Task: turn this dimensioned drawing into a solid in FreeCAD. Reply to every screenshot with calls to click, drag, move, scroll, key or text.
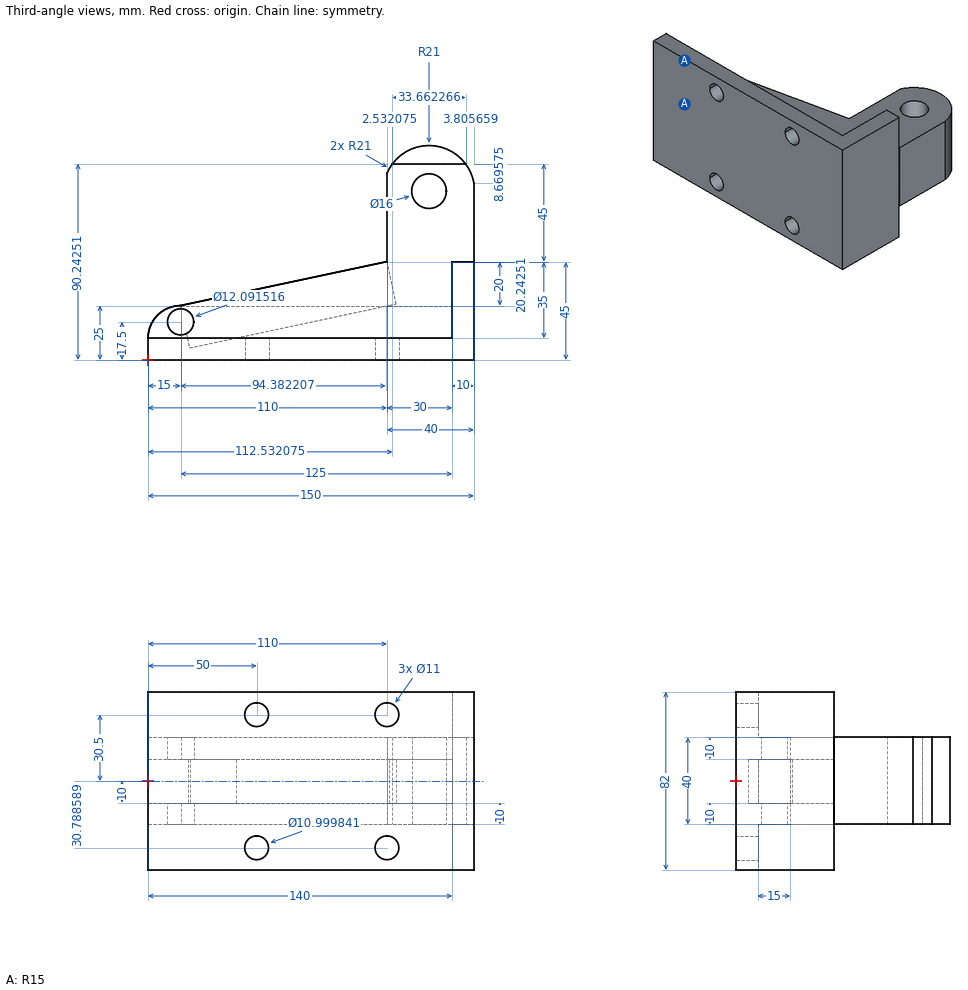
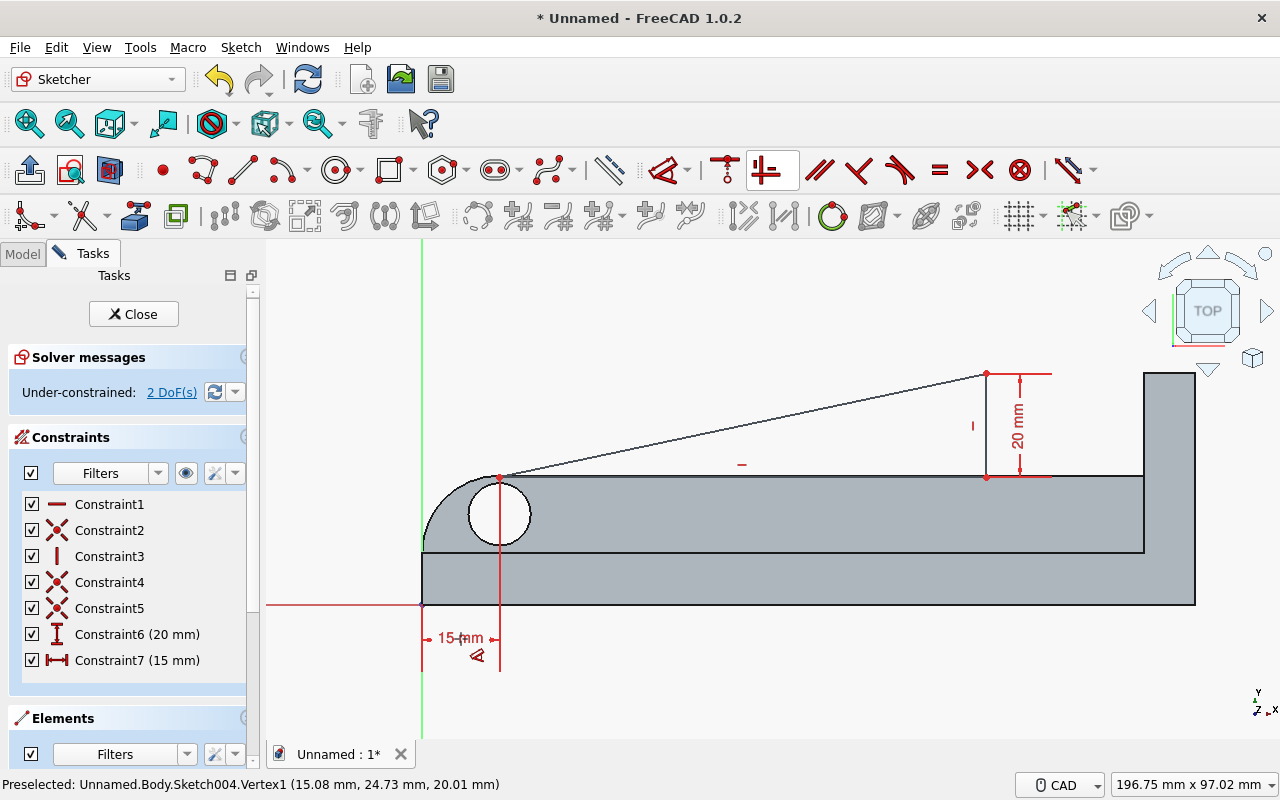
click(500, 477)
click(388, 541)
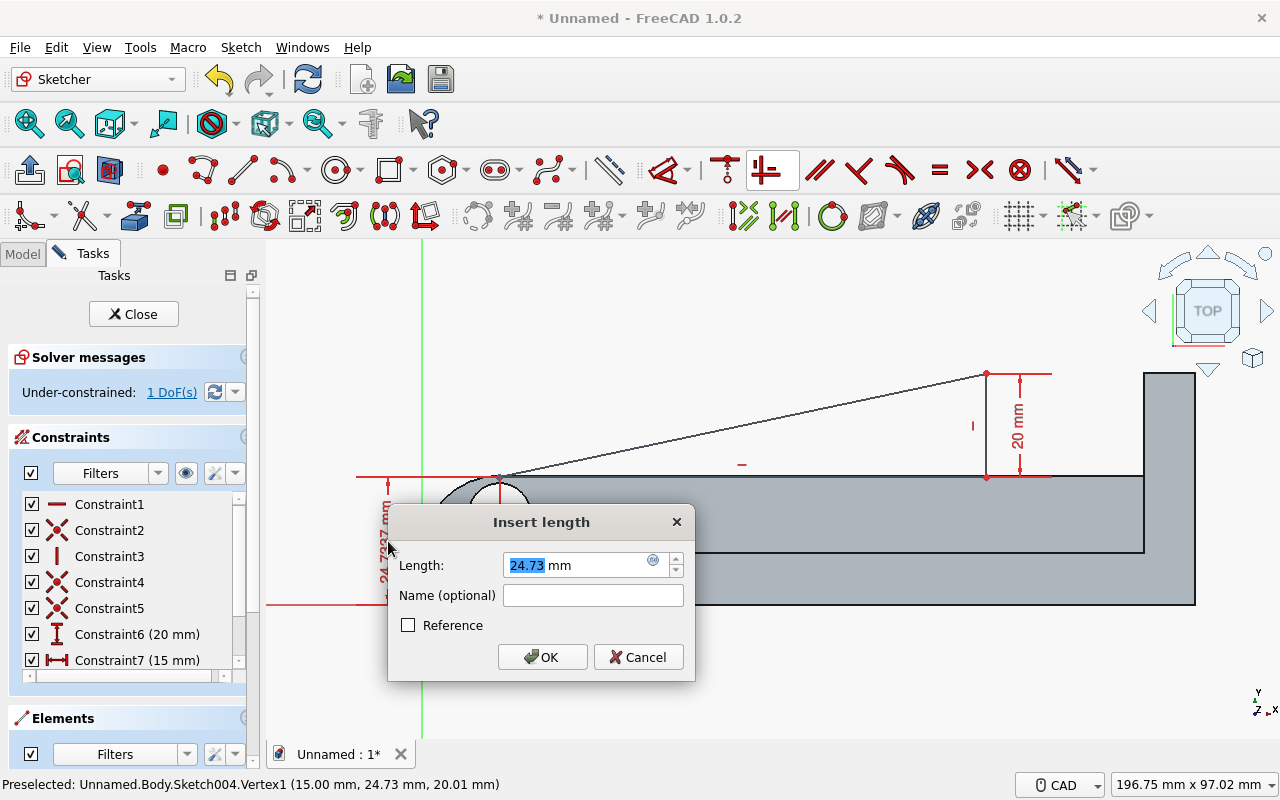
text(25)
key(Return)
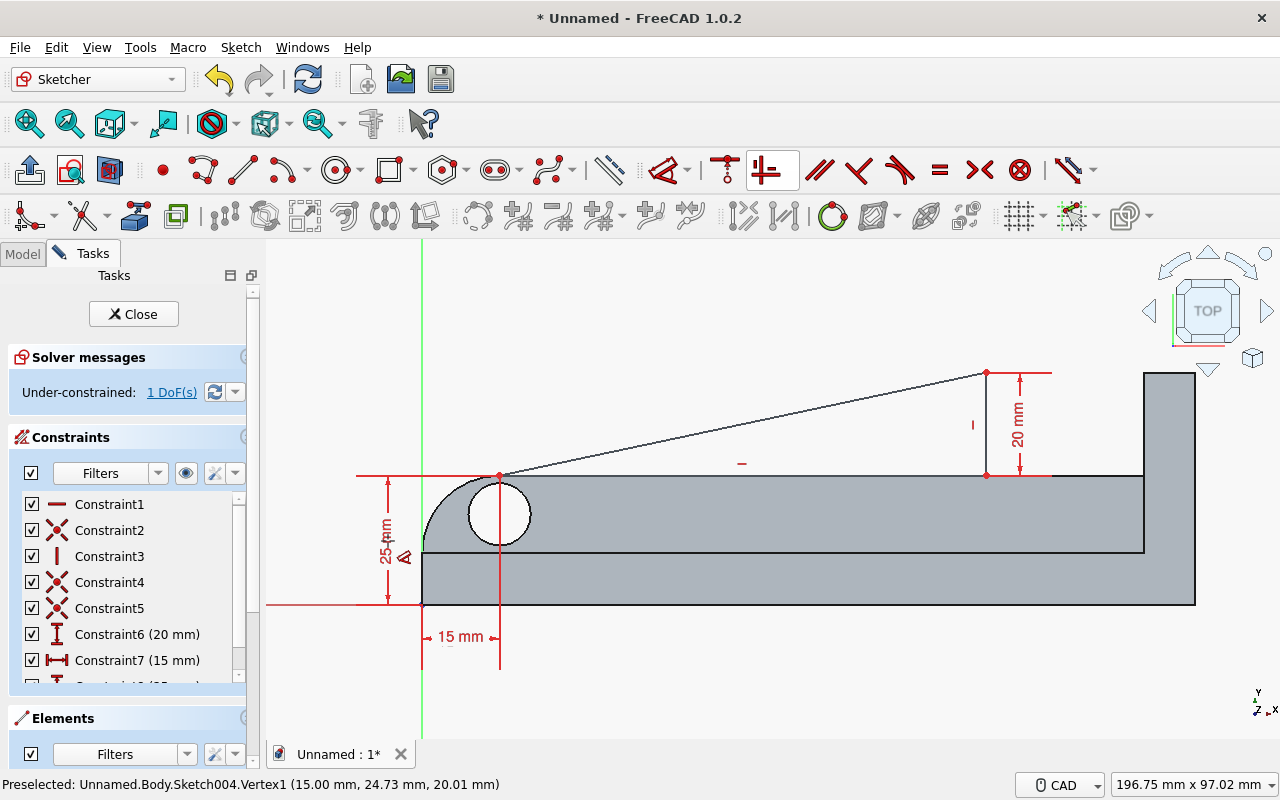
click(645, 476)
click(743, 442)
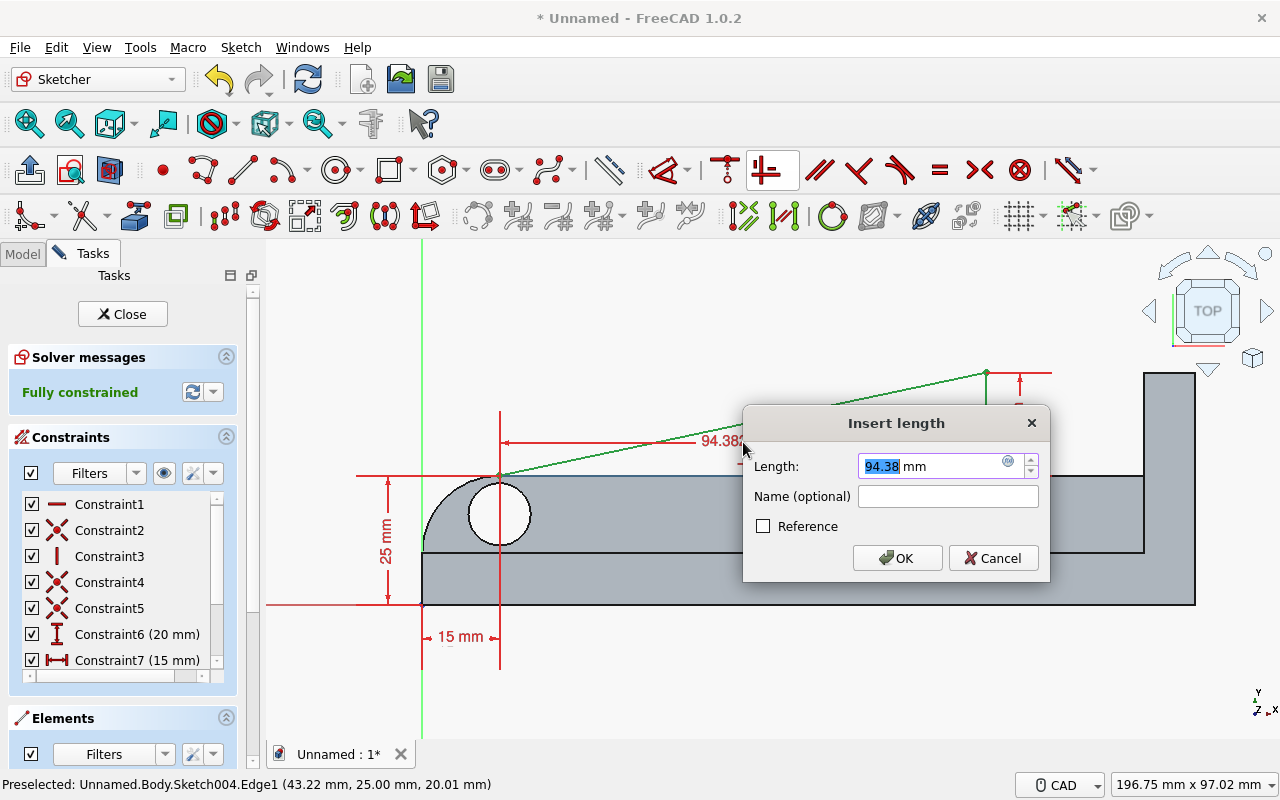
text(94.382207)
key(Return)
key(Escape)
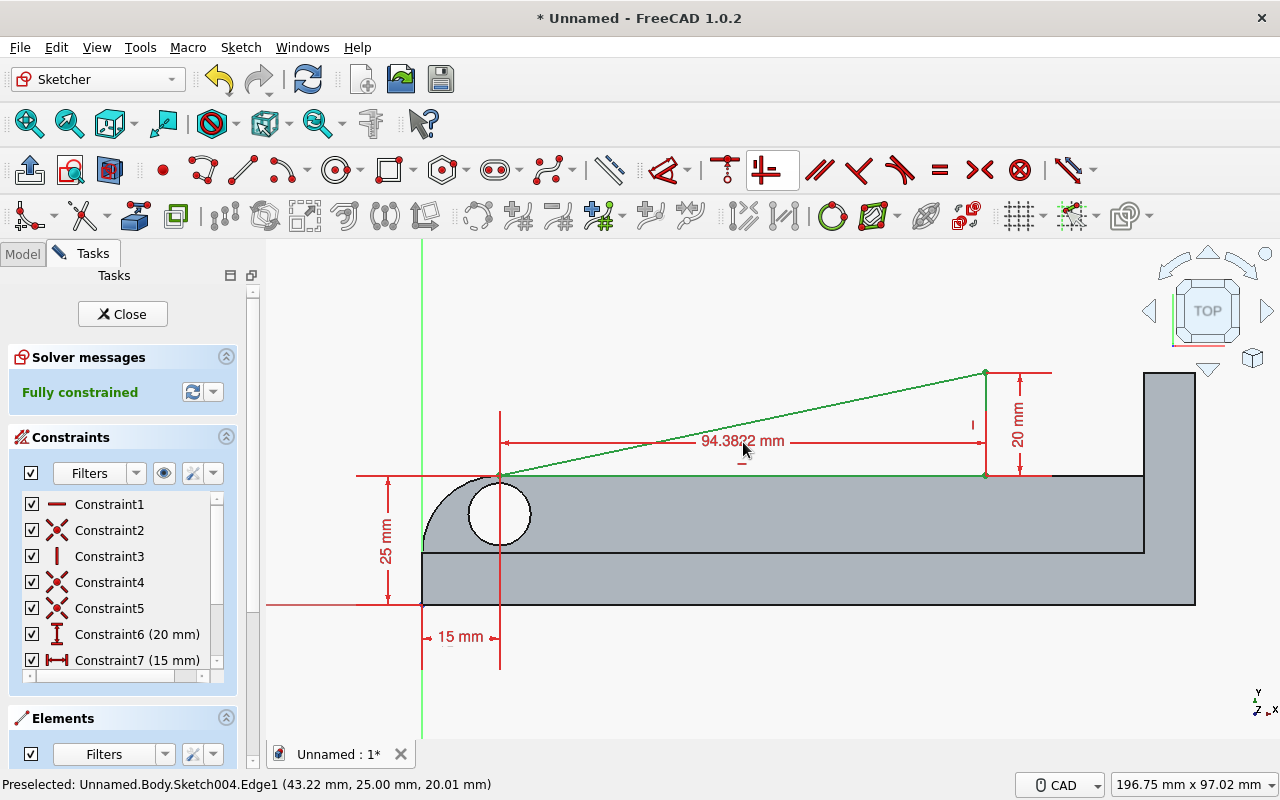
click(123, 314)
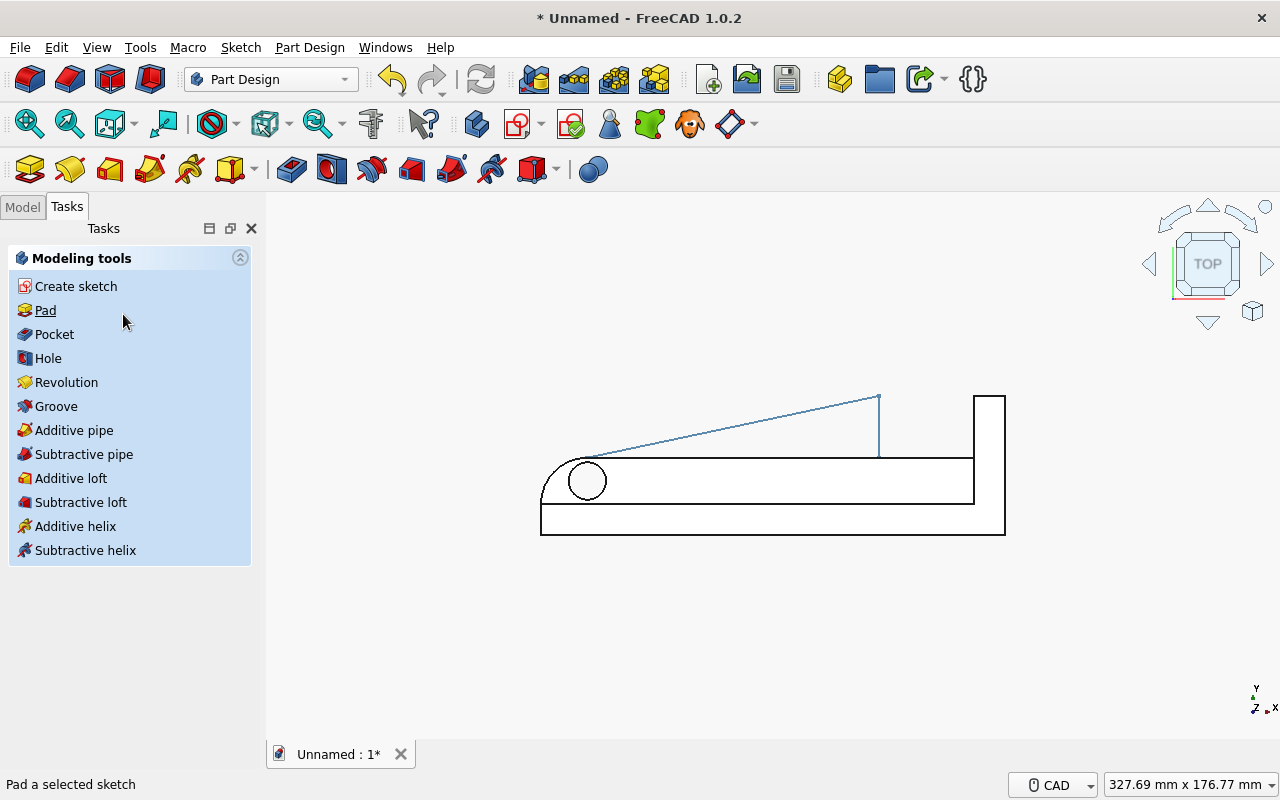
click(30, 170)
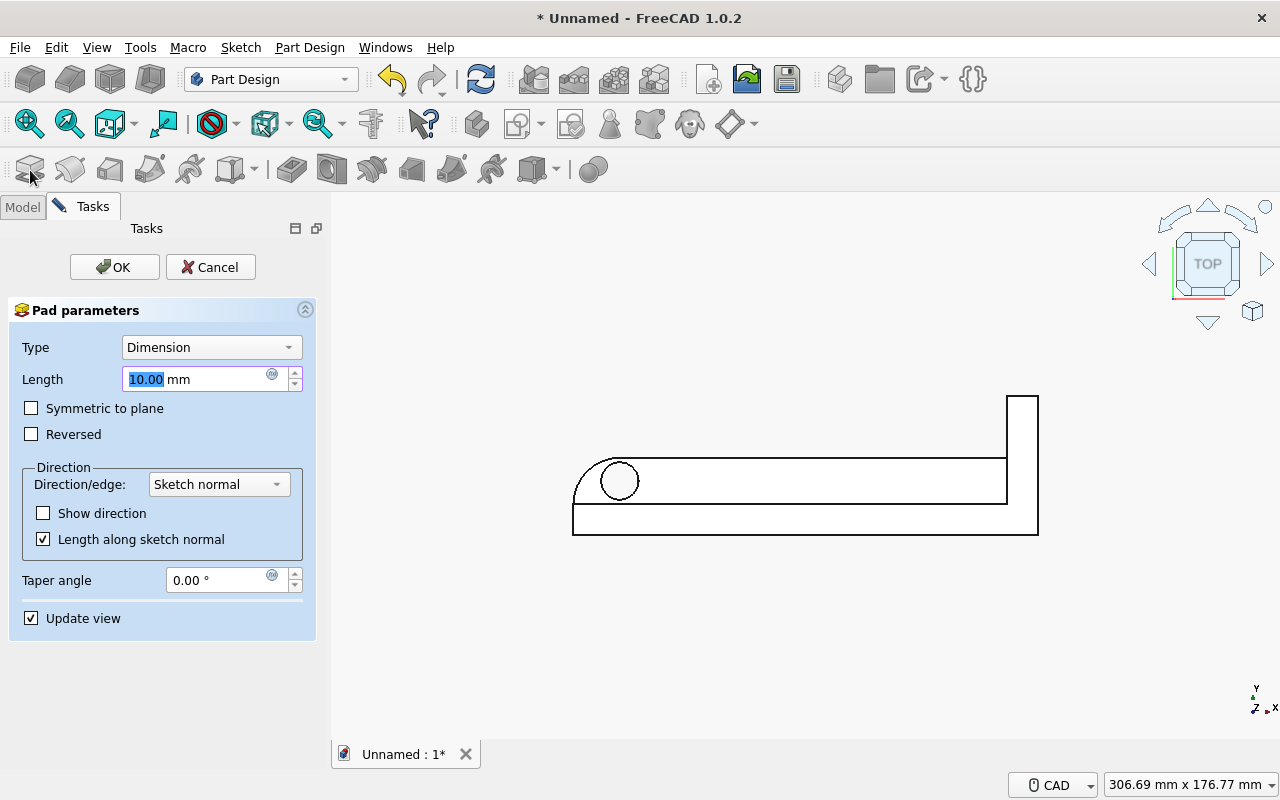
text(10)
key(Tab)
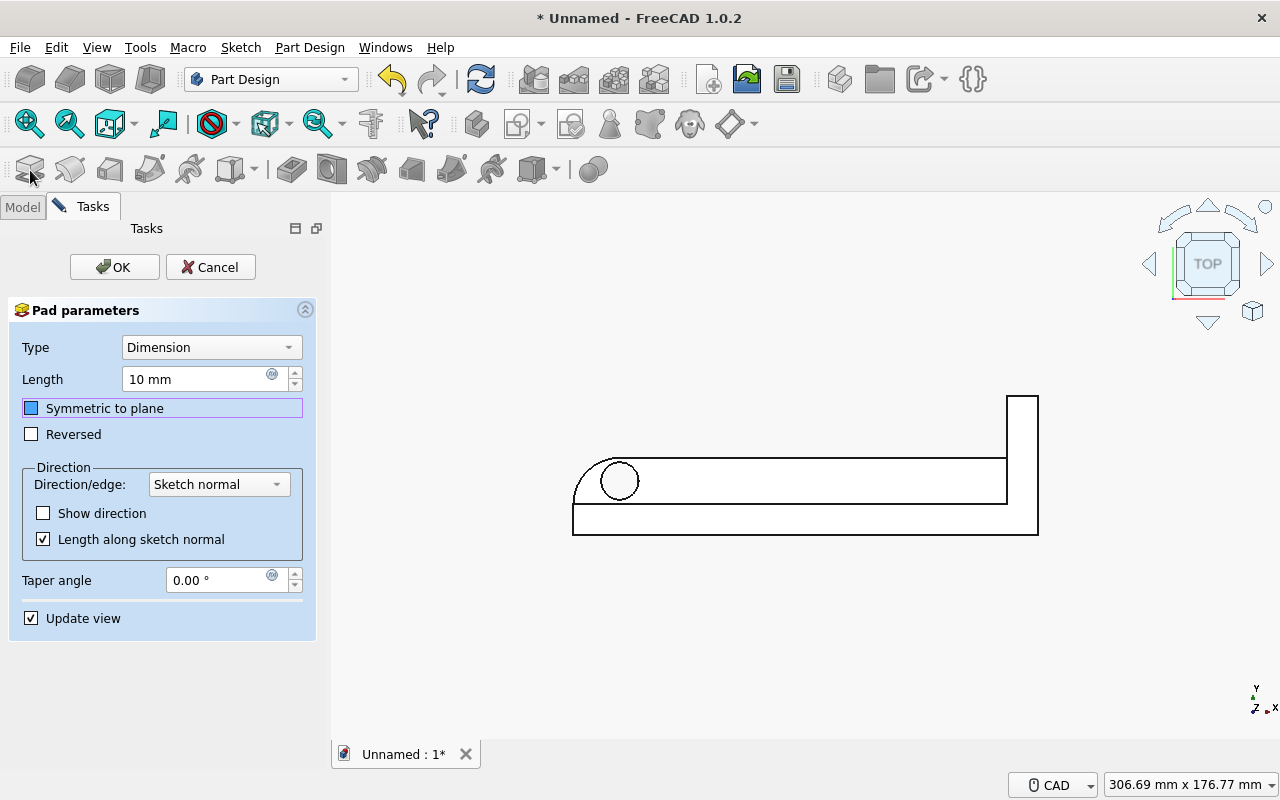
click(30, 434)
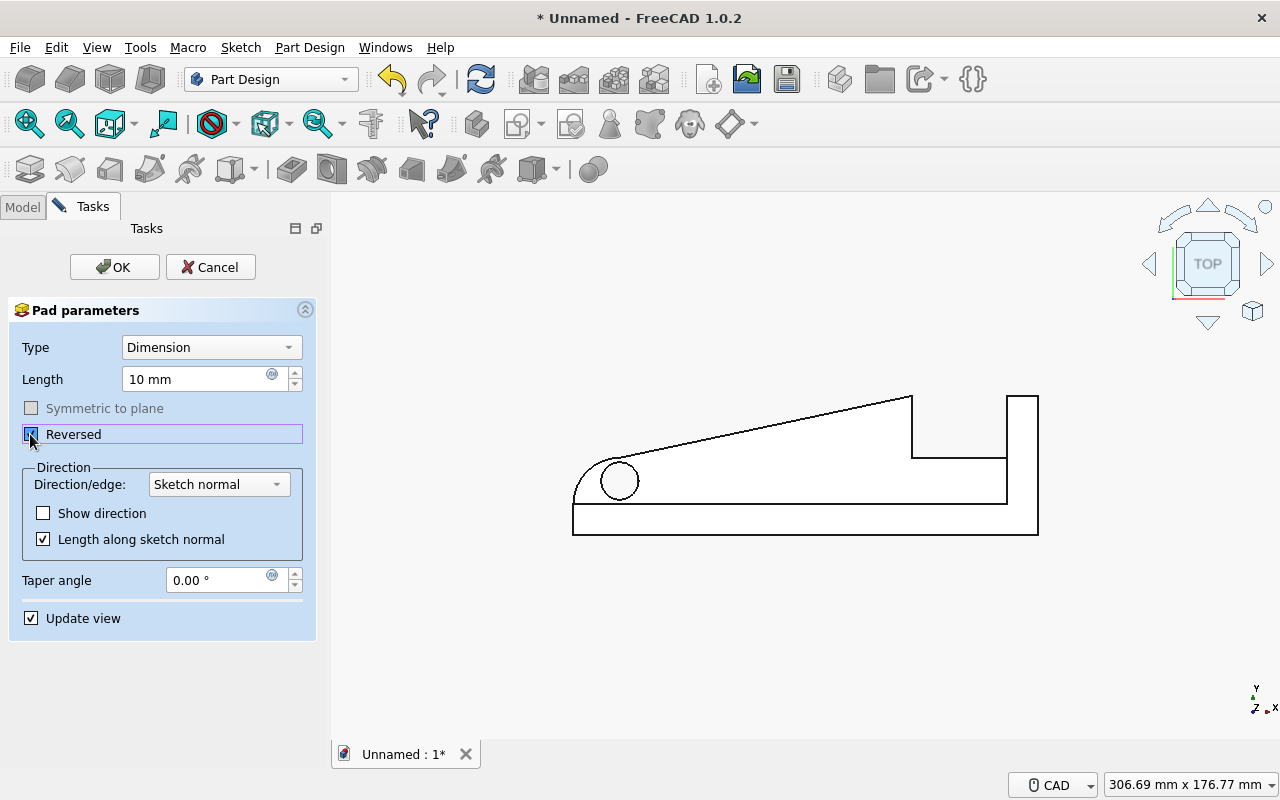
click(115, 267)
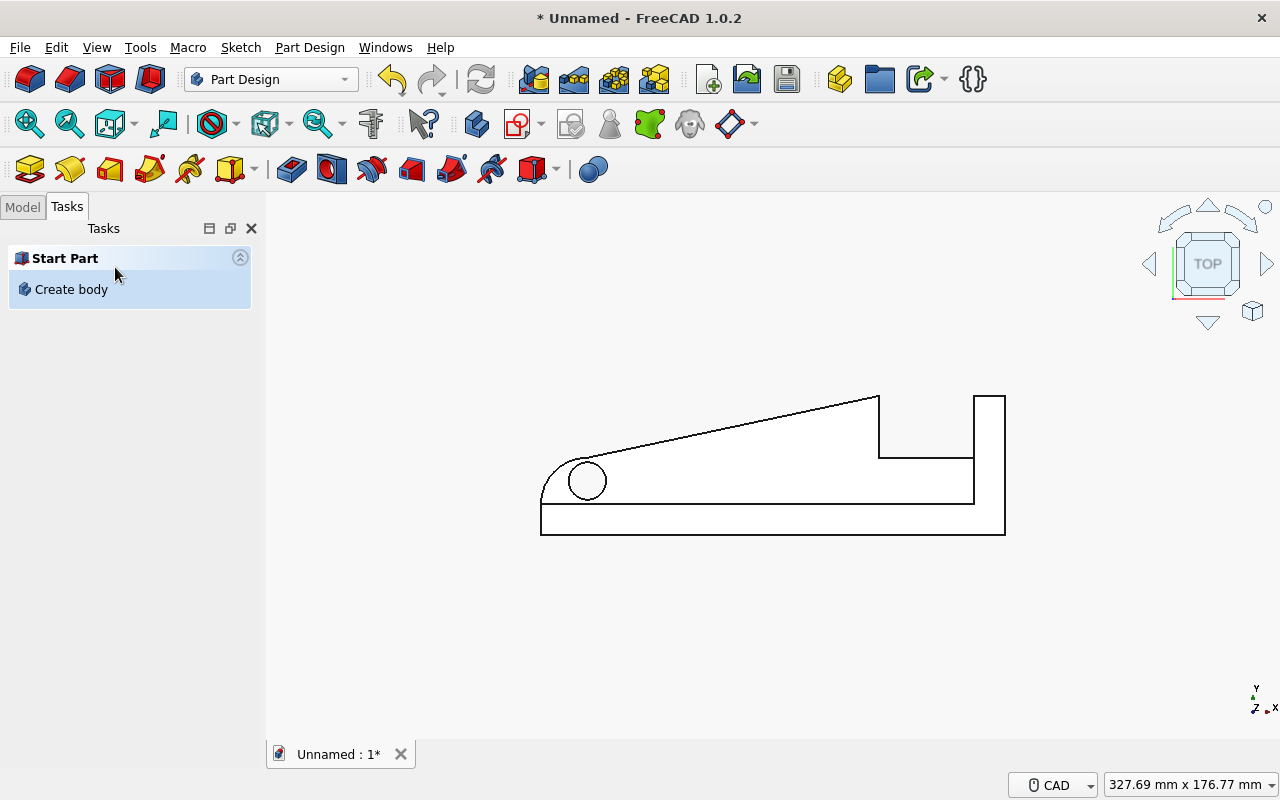
key(5)